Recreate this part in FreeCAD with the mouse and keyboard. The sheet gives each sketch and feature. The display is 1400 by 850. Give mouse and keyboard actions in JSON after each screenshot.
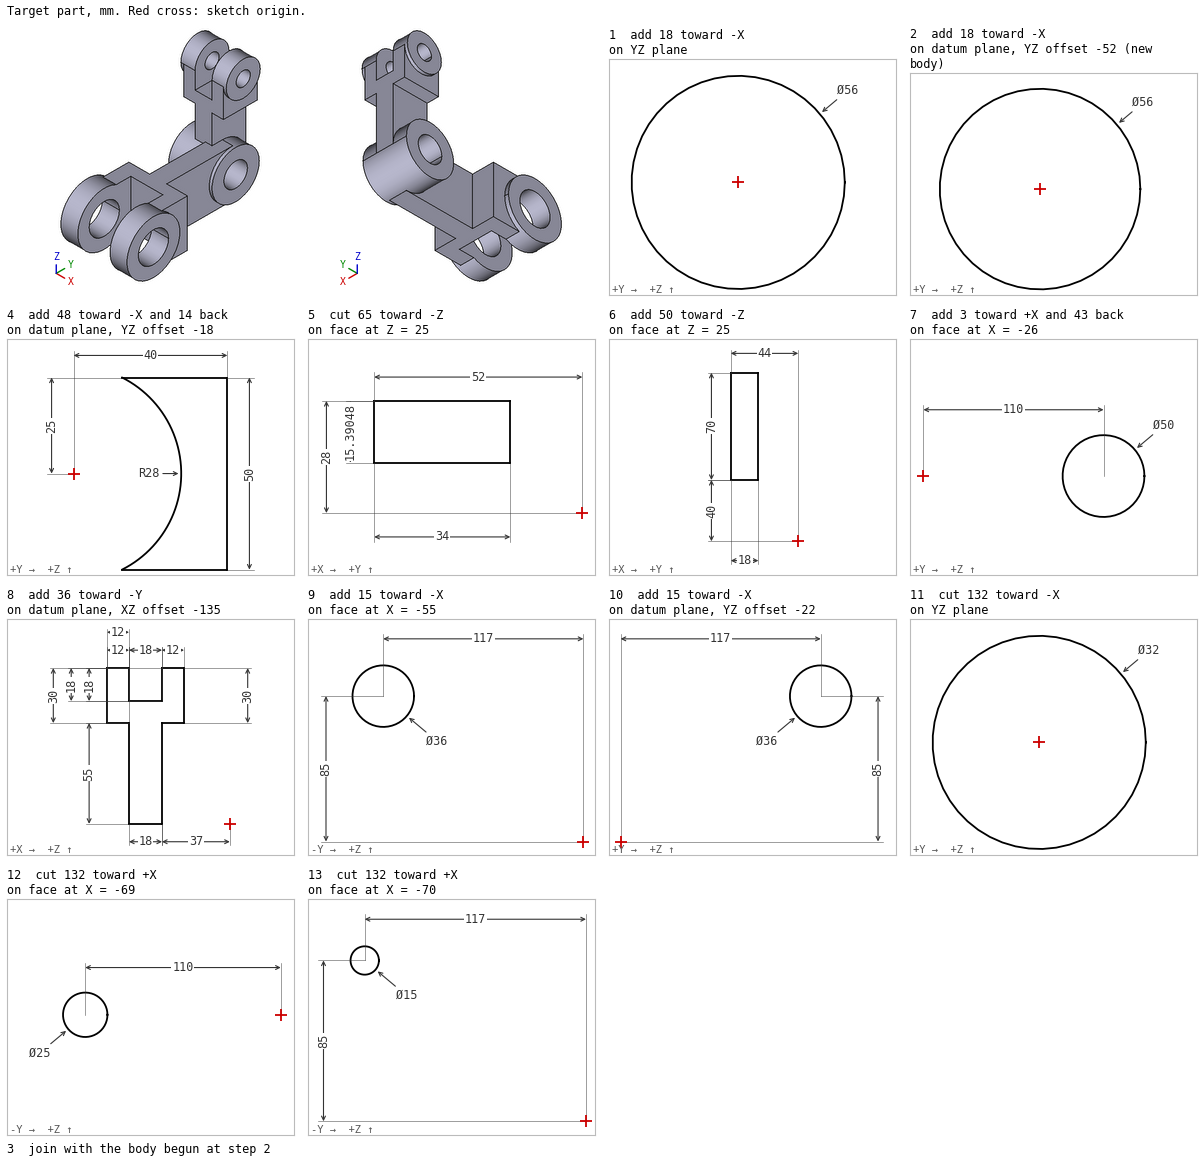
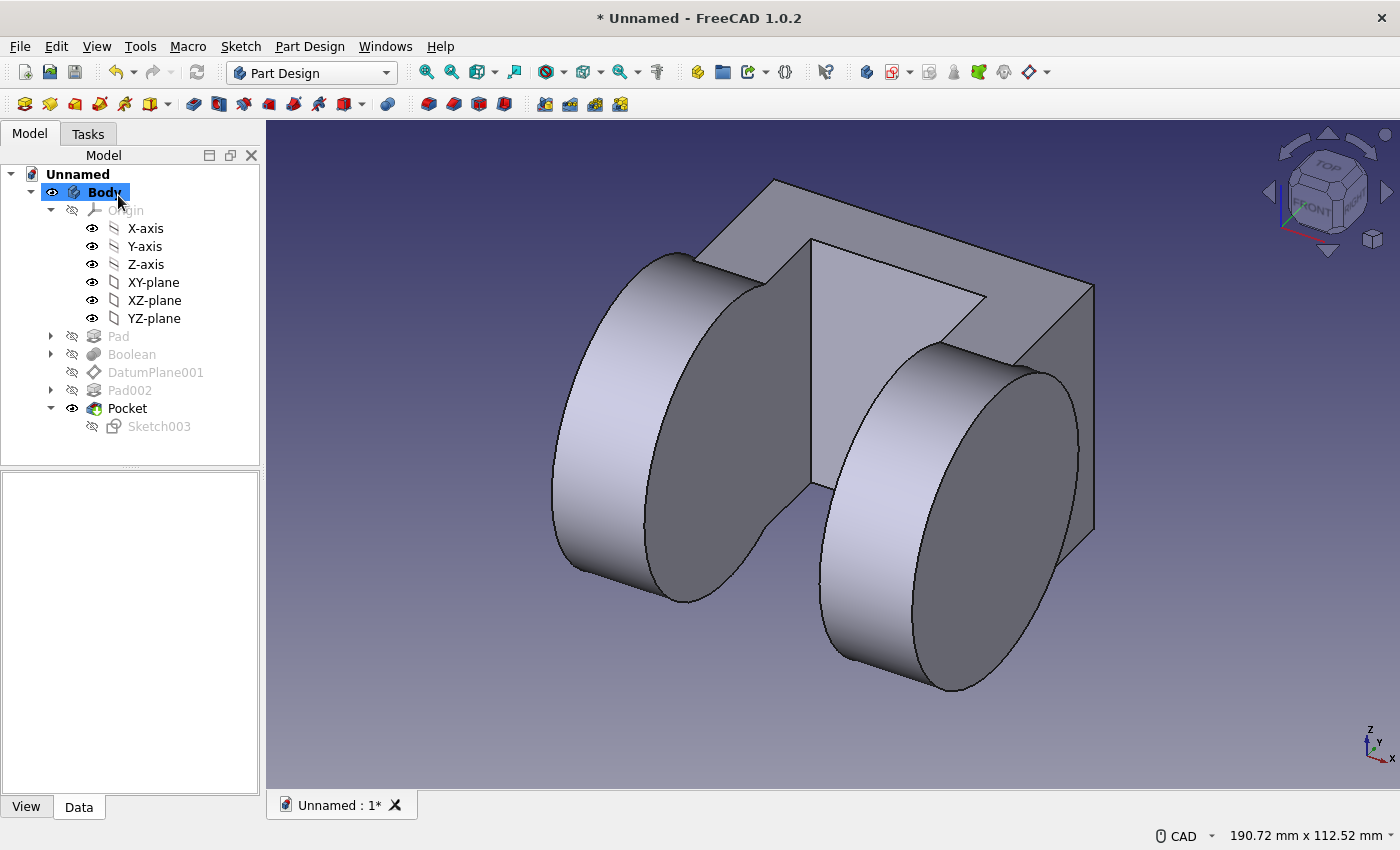
{"action": "left_click", "coordinate": [1008, 279]}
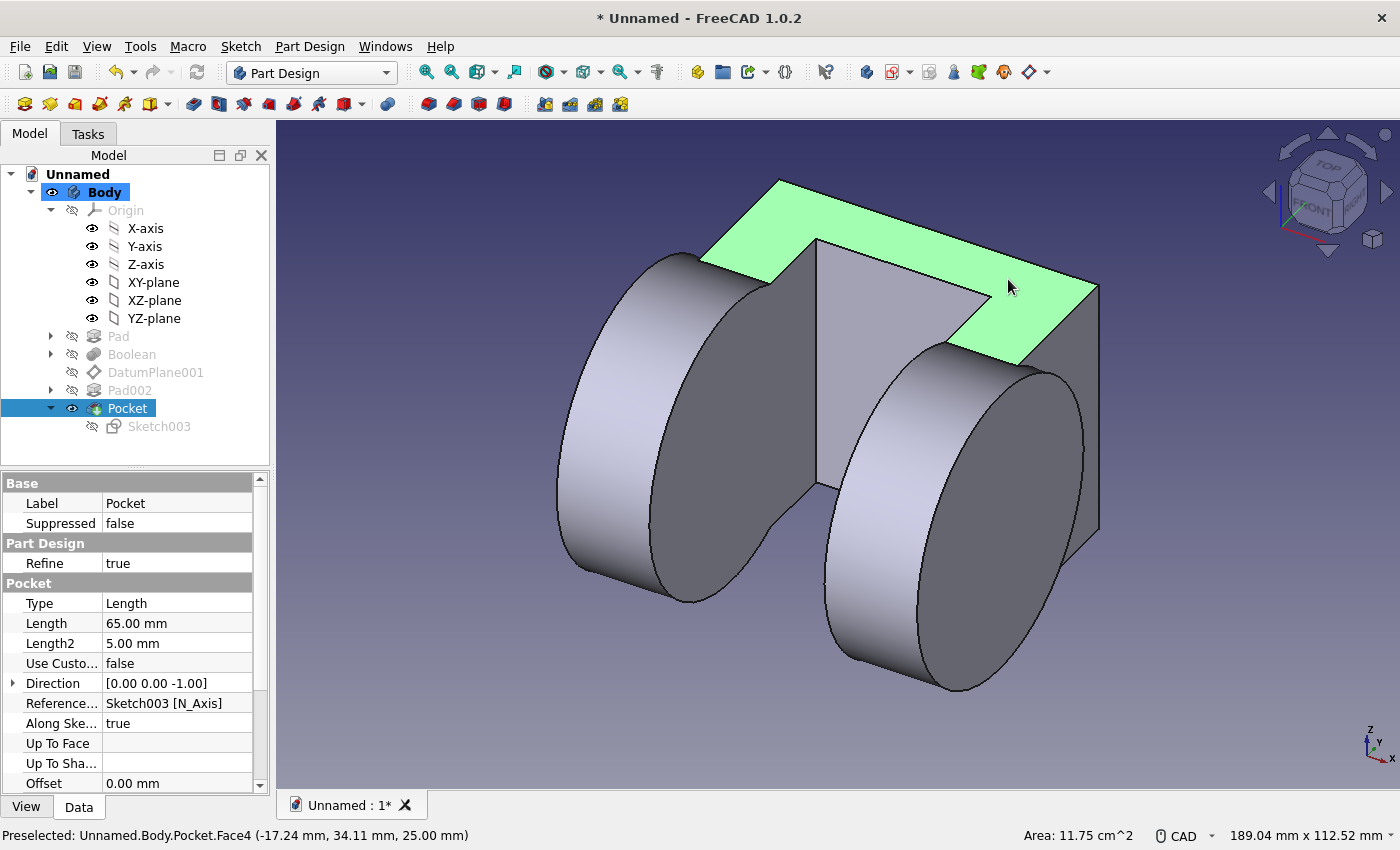
{"action": "left_click", "coordinate": [892, 72]}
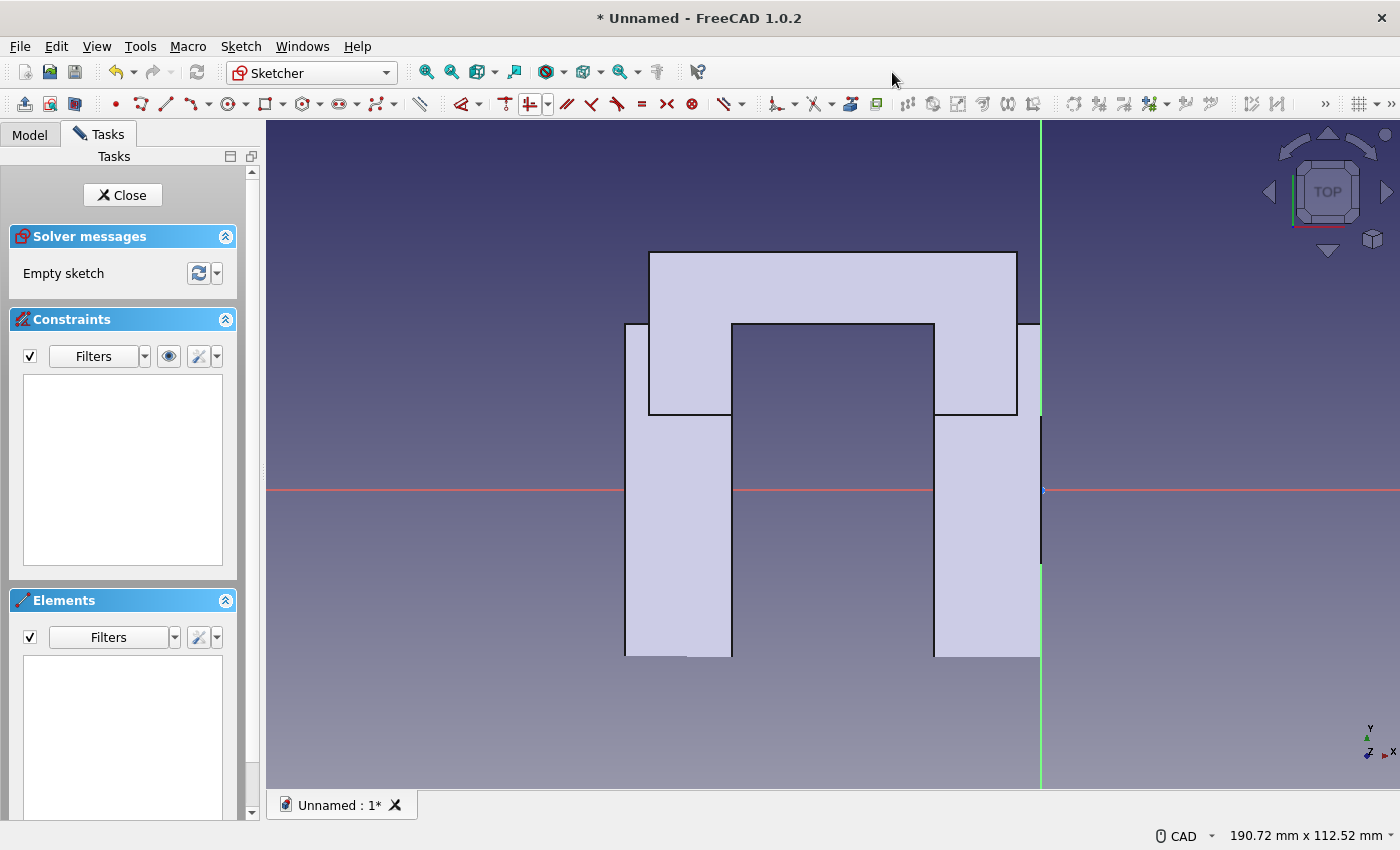
{"action": "scroll", "coordinate": [587, 761], "scroll_direction": "down", "scroll_amount": 3}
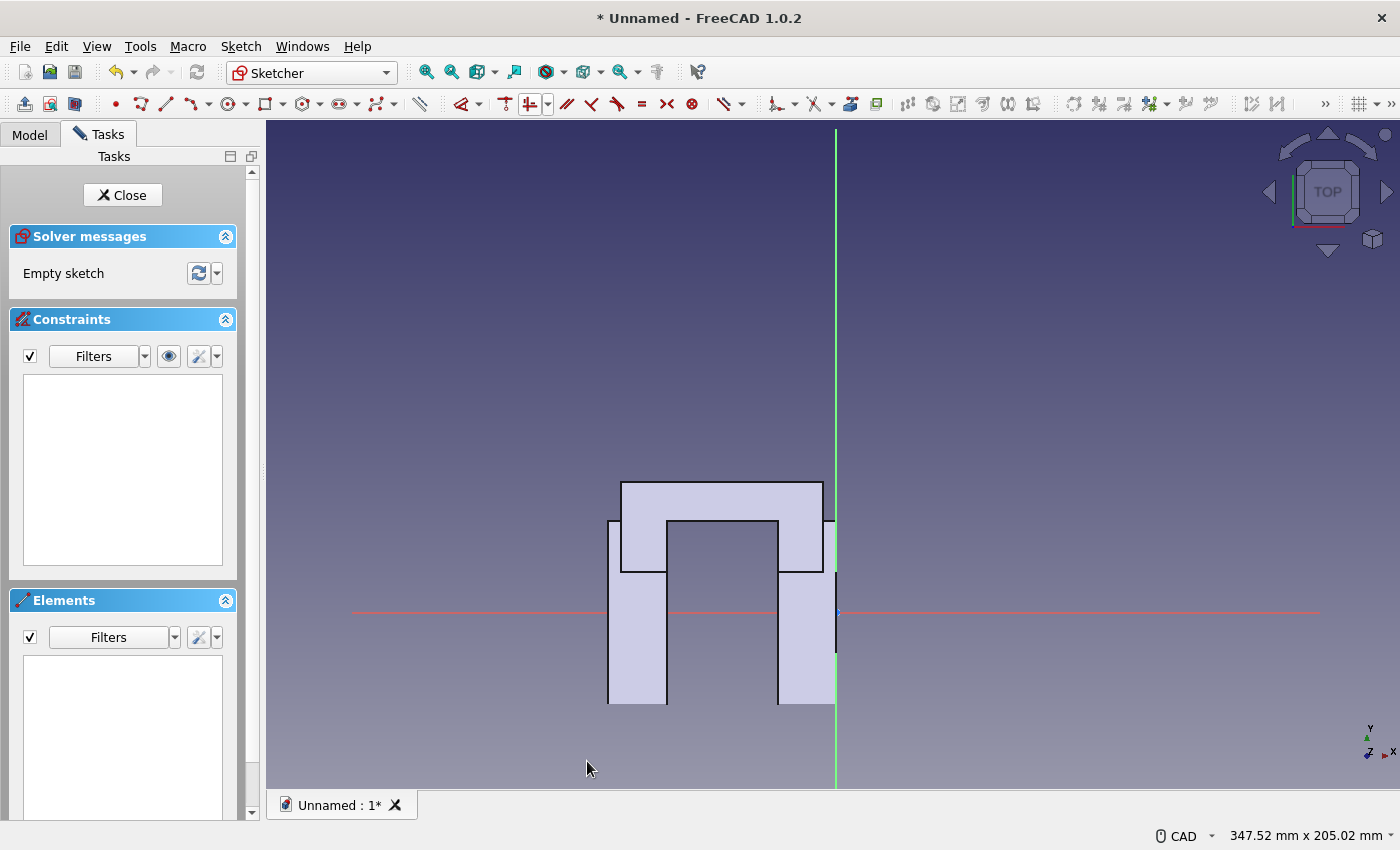
{"action": "left_click", "coordinate": [264, 104]}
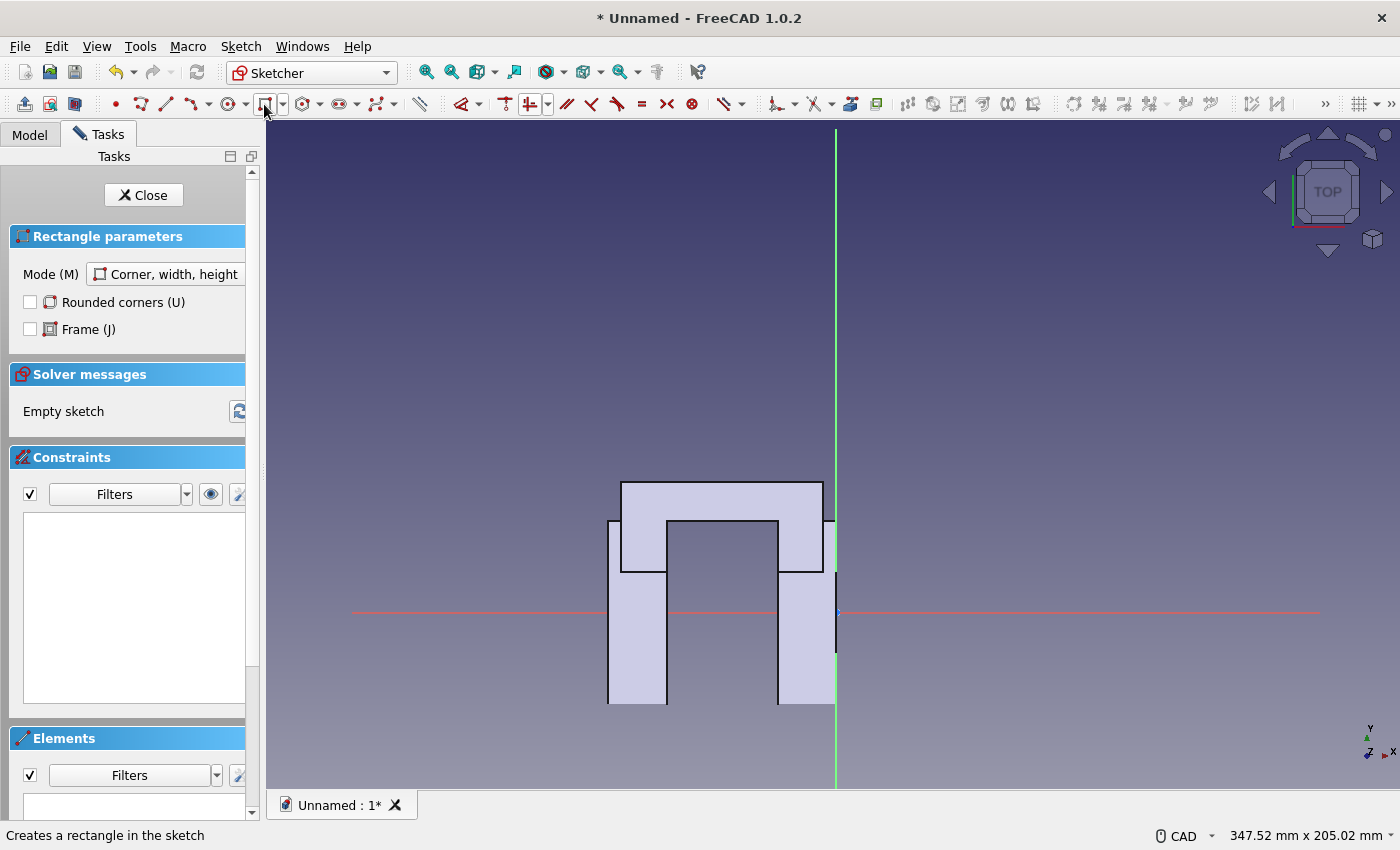
{"action": "left_click", "coordinate": [693, 254]}
{"action": "left_click", "coordinate": [752, 482]}
{"action": "key", "text": "Escape"}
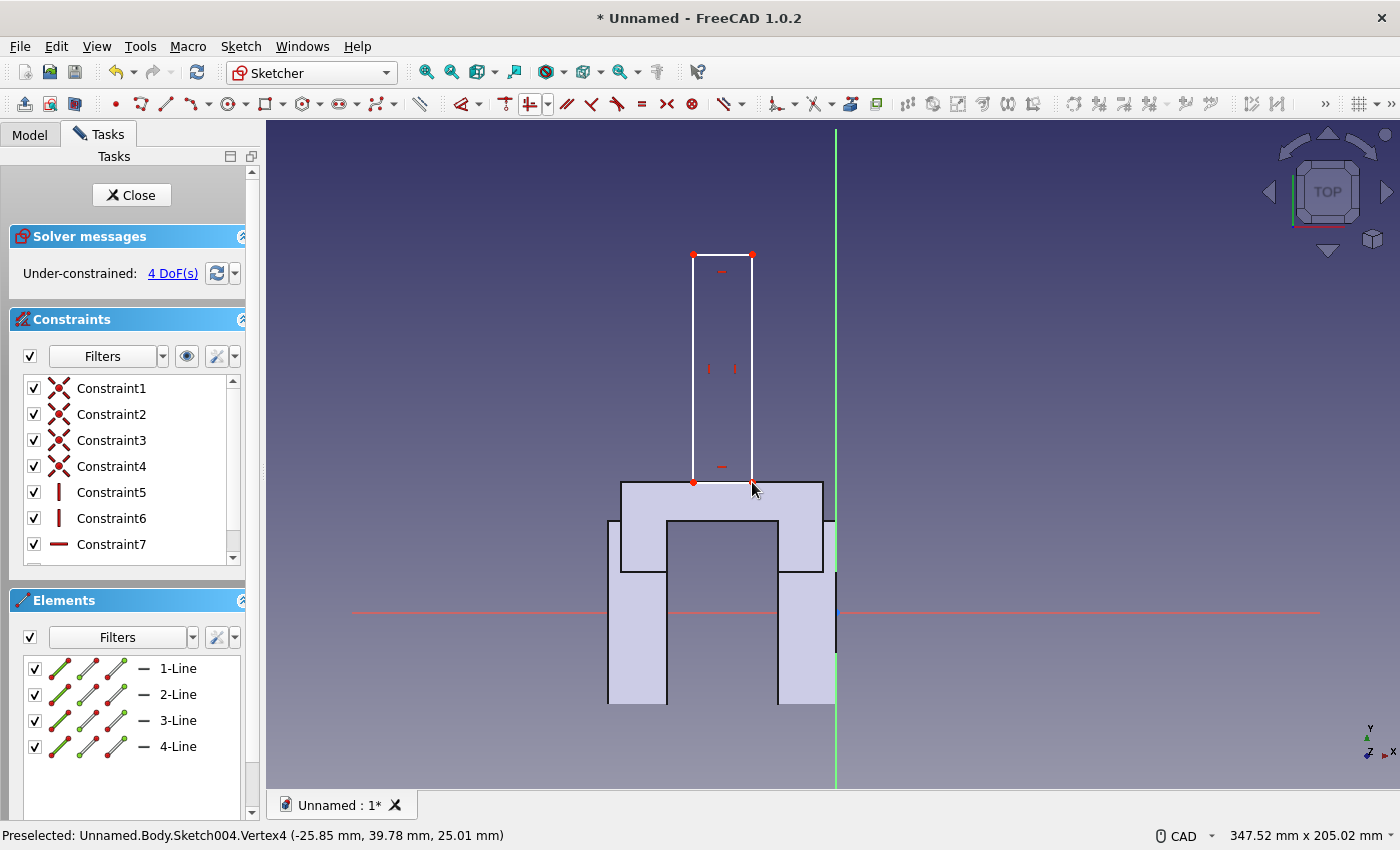
{"action": "left_click", "coordinate": [693, 323]}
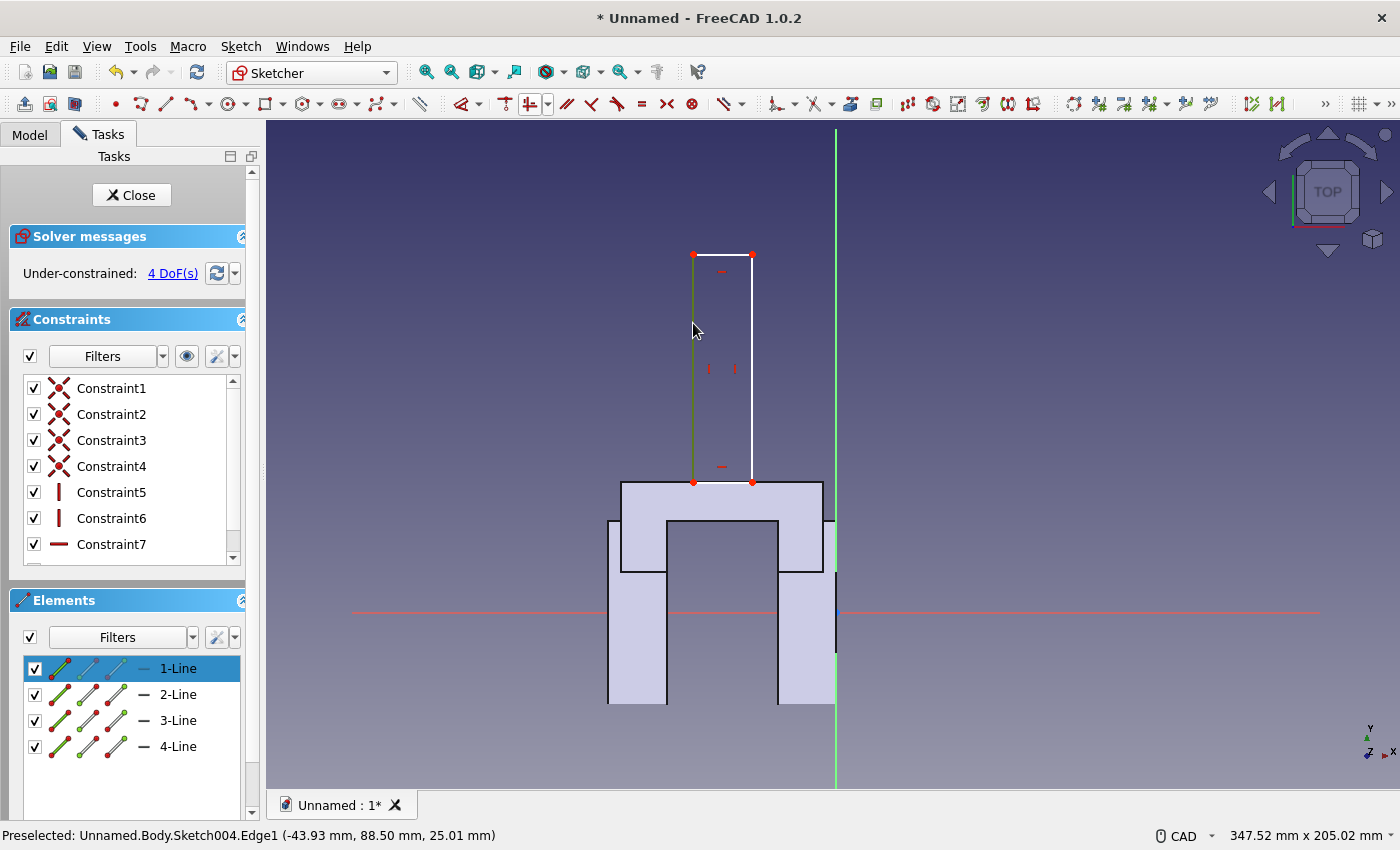
{"action": "key", "text": "i"}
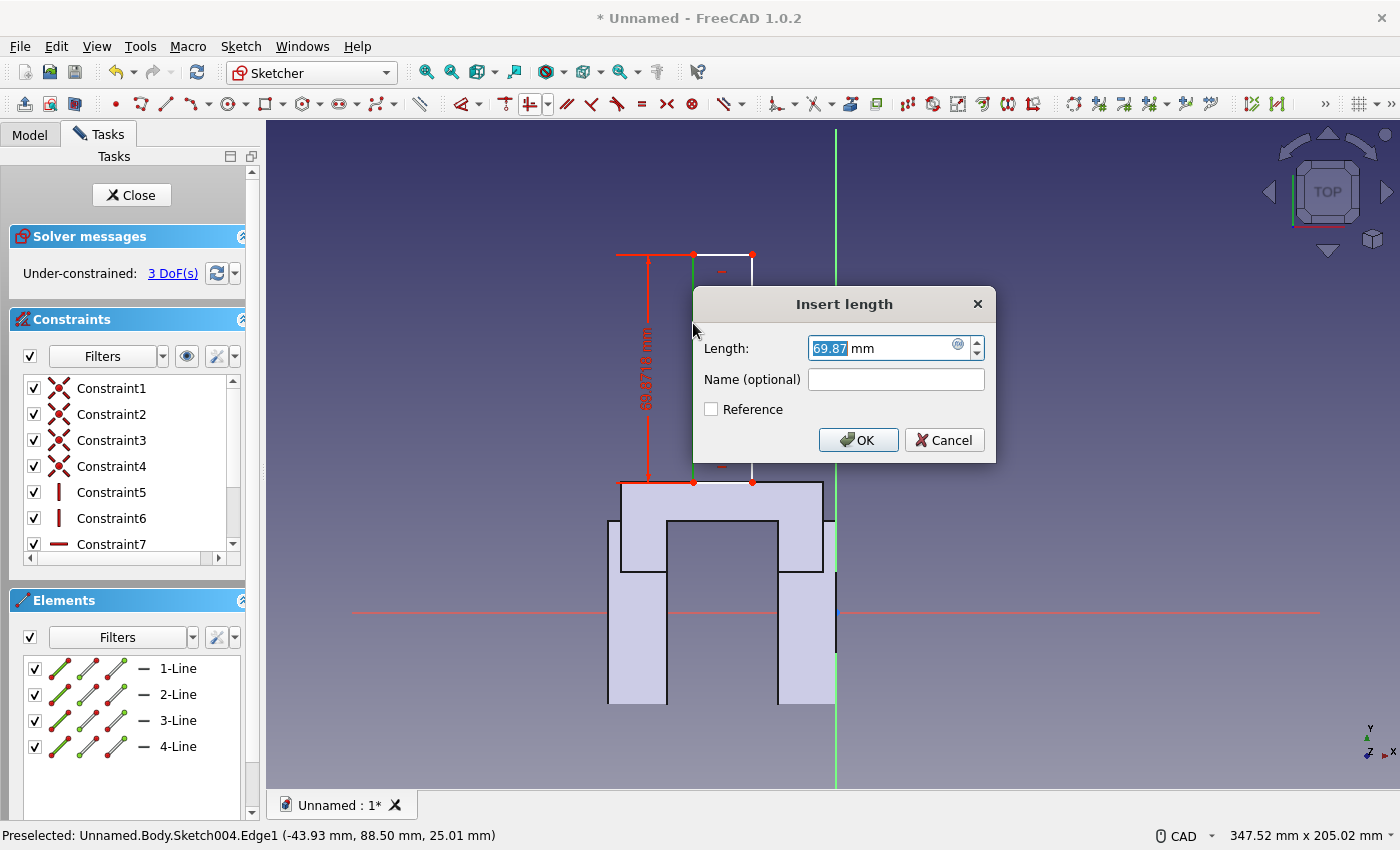
{"action": "type", "text": "70"}
{"action": "key", "text": "Return"}